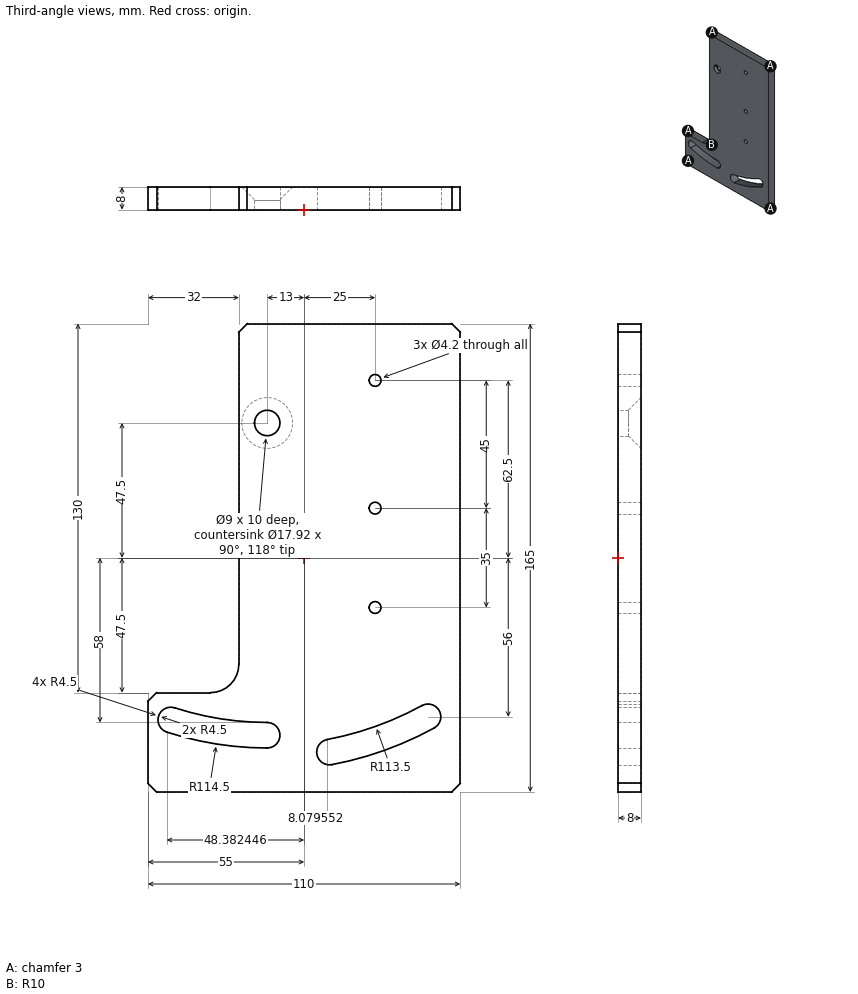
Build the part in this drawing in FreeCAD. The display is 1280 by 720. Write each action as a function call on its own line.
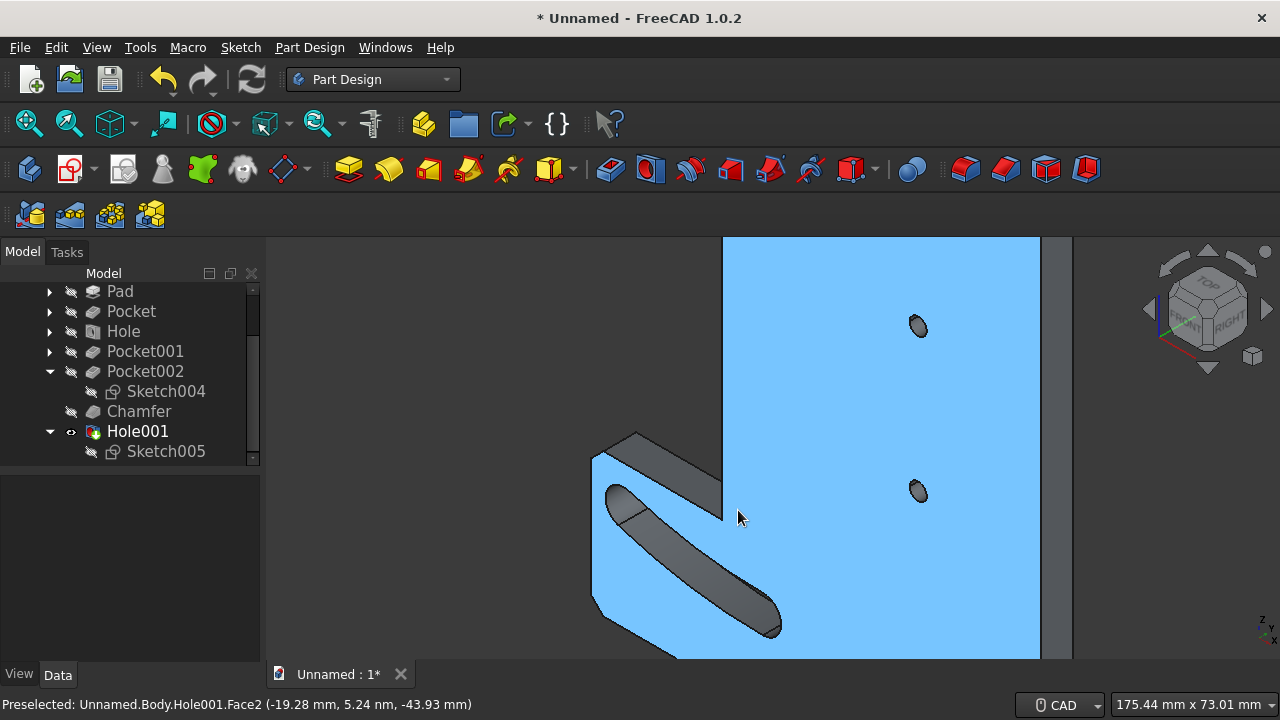
click(30, 124)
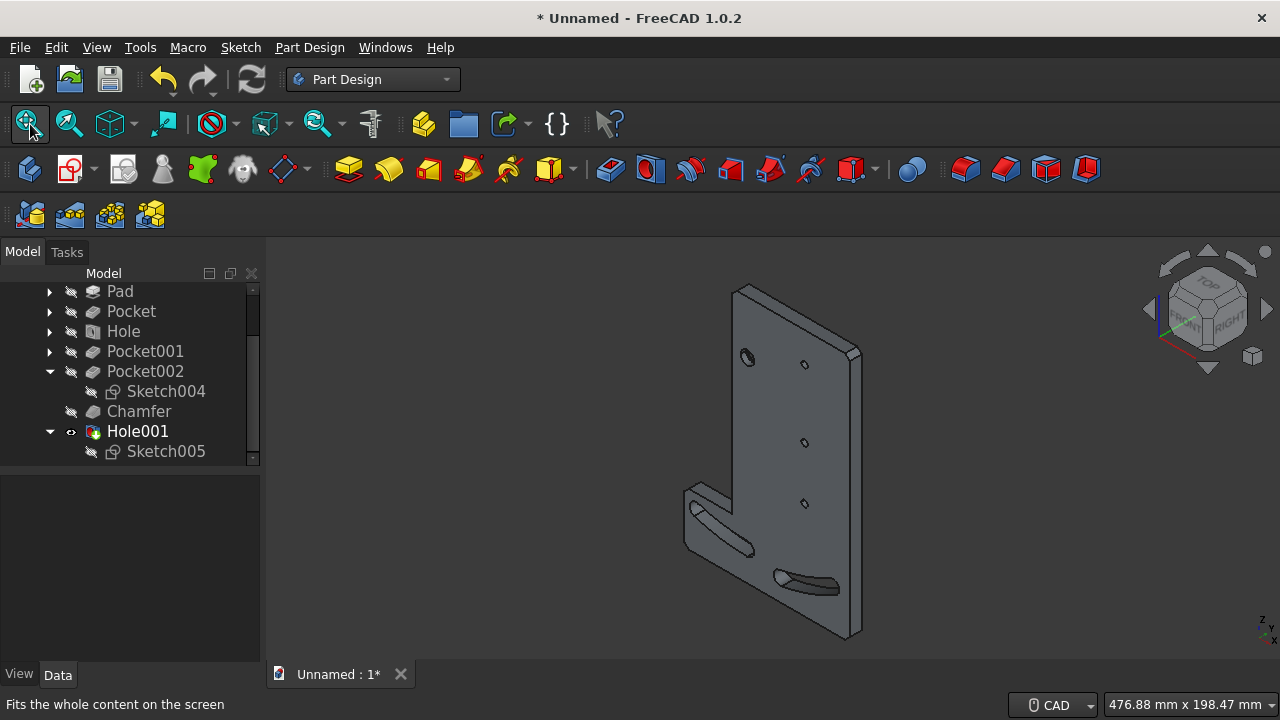
key(2)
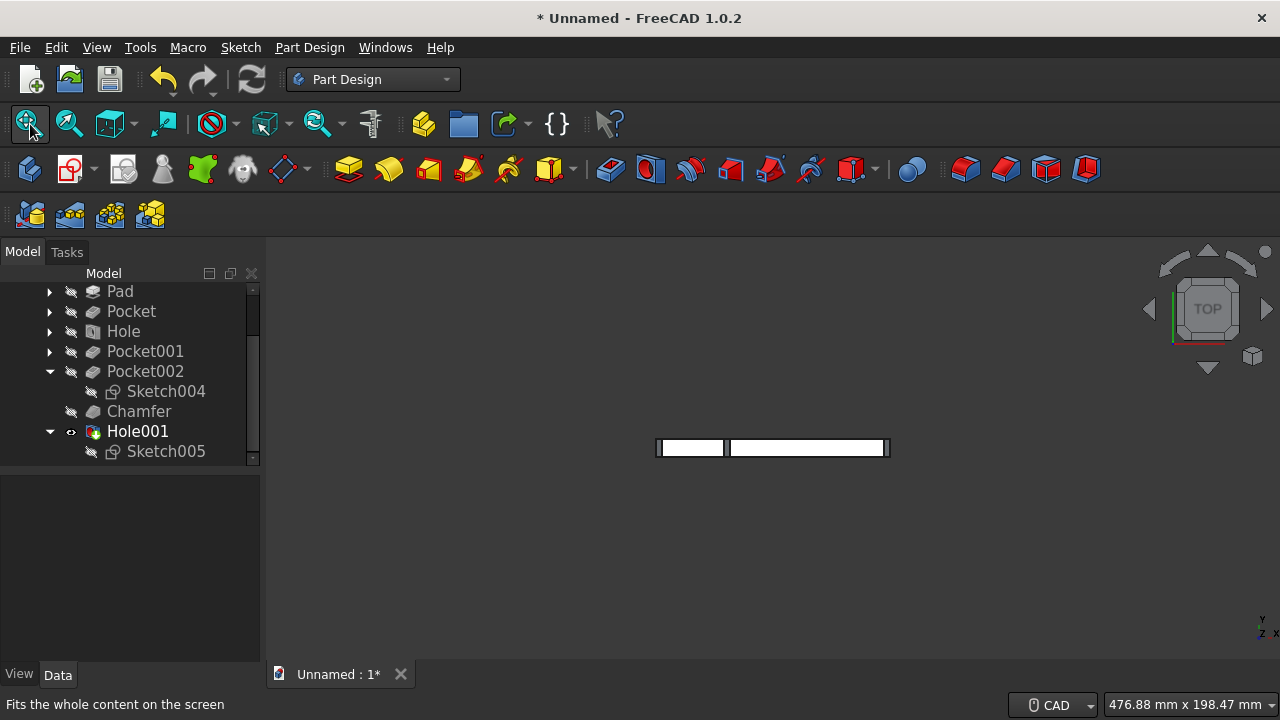
click(30, 124)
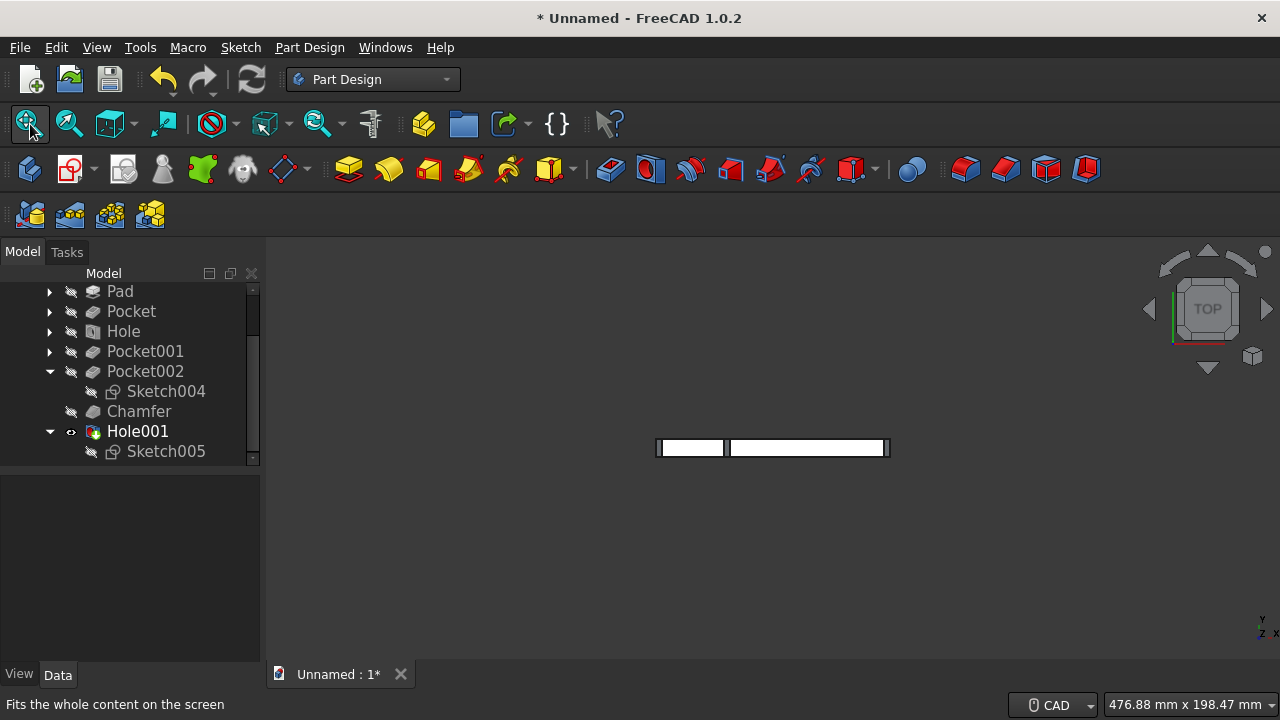
scroll(724, 447, up, 5)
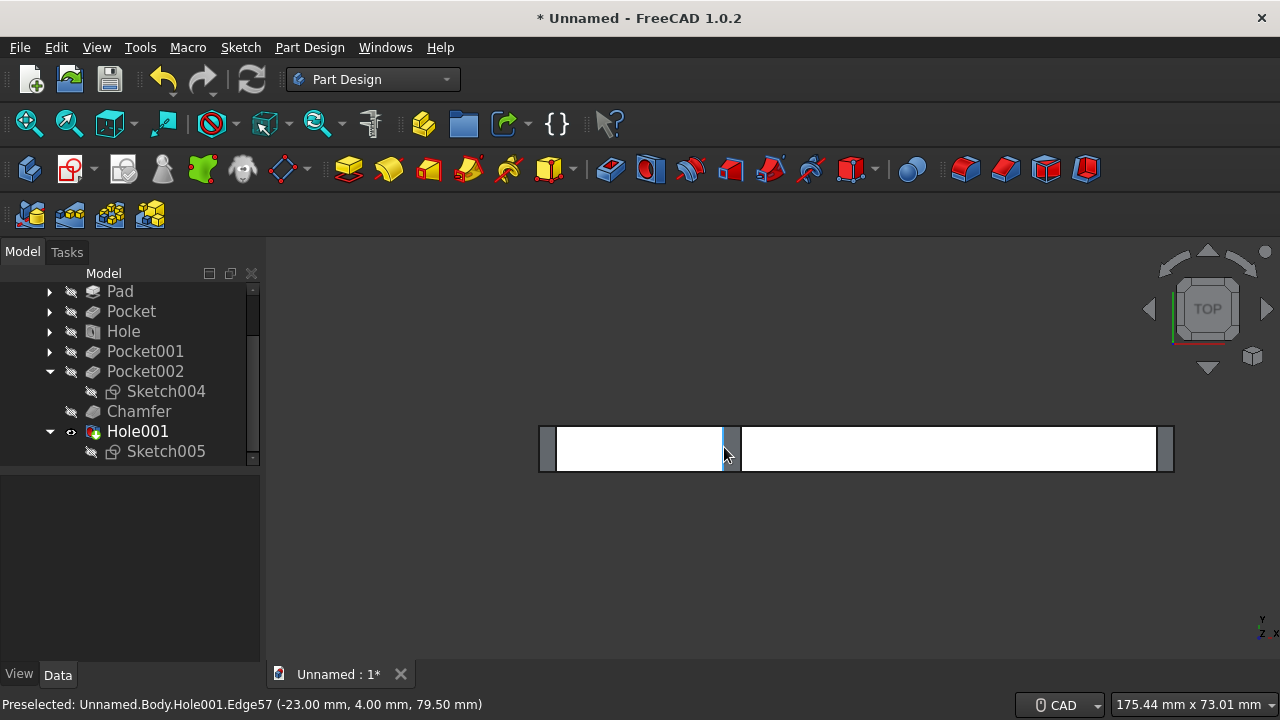
click(30, 124)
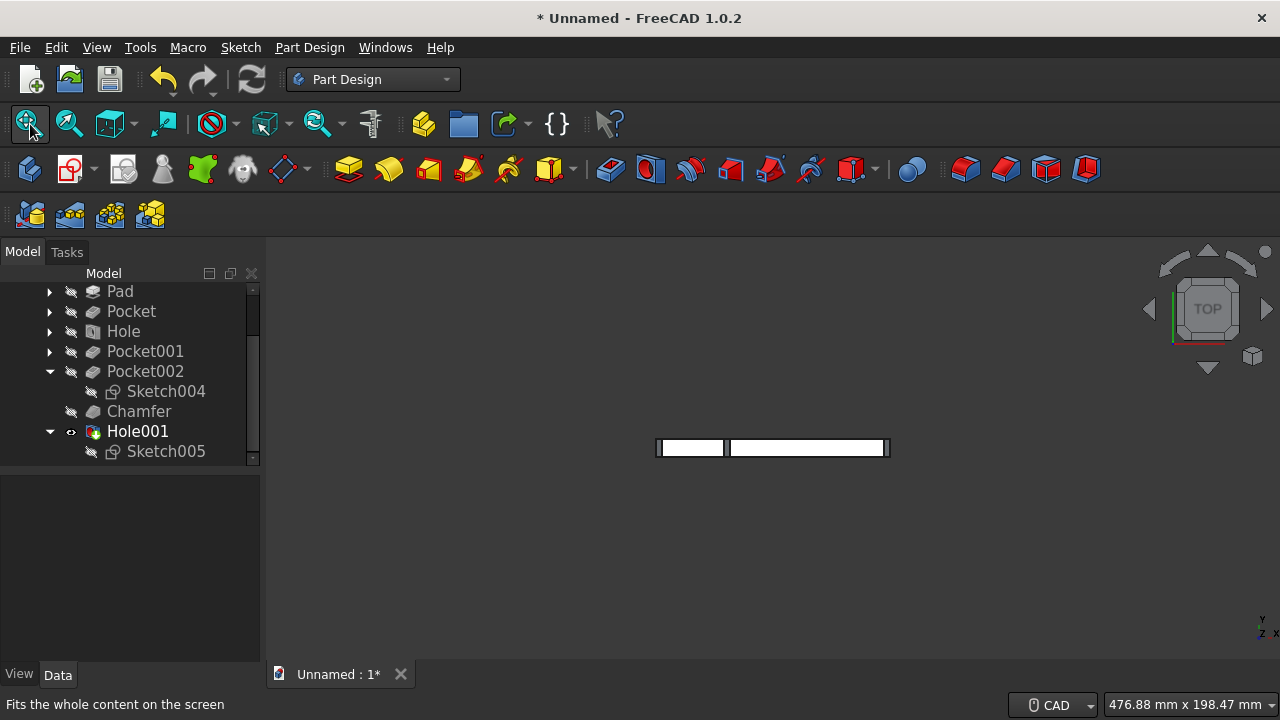
key(1)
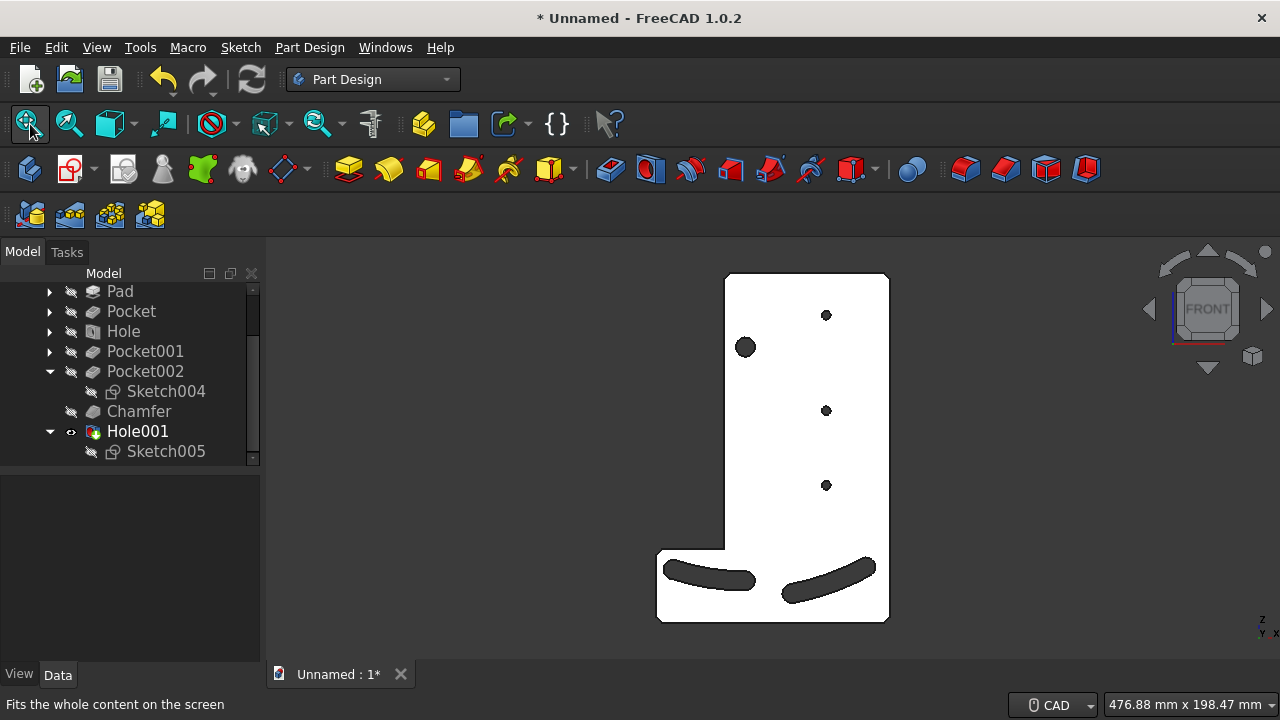
scroll(724, 548, up, 5)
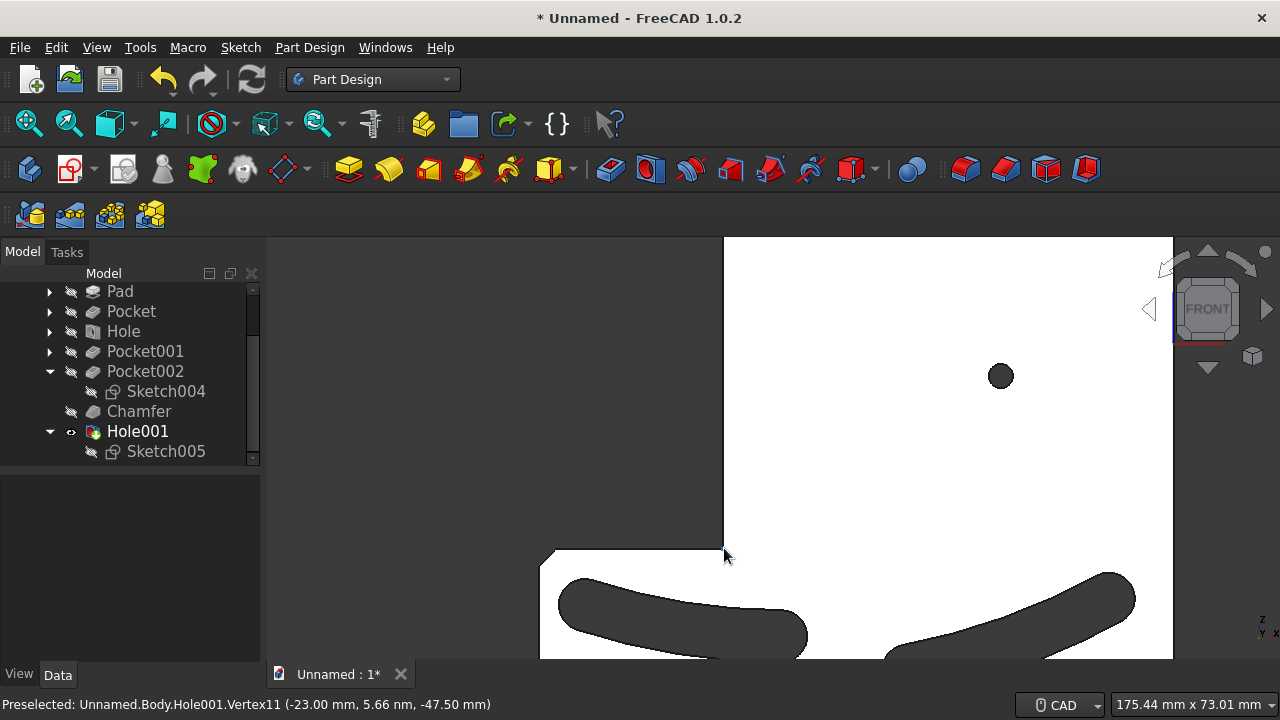
click(30, 124)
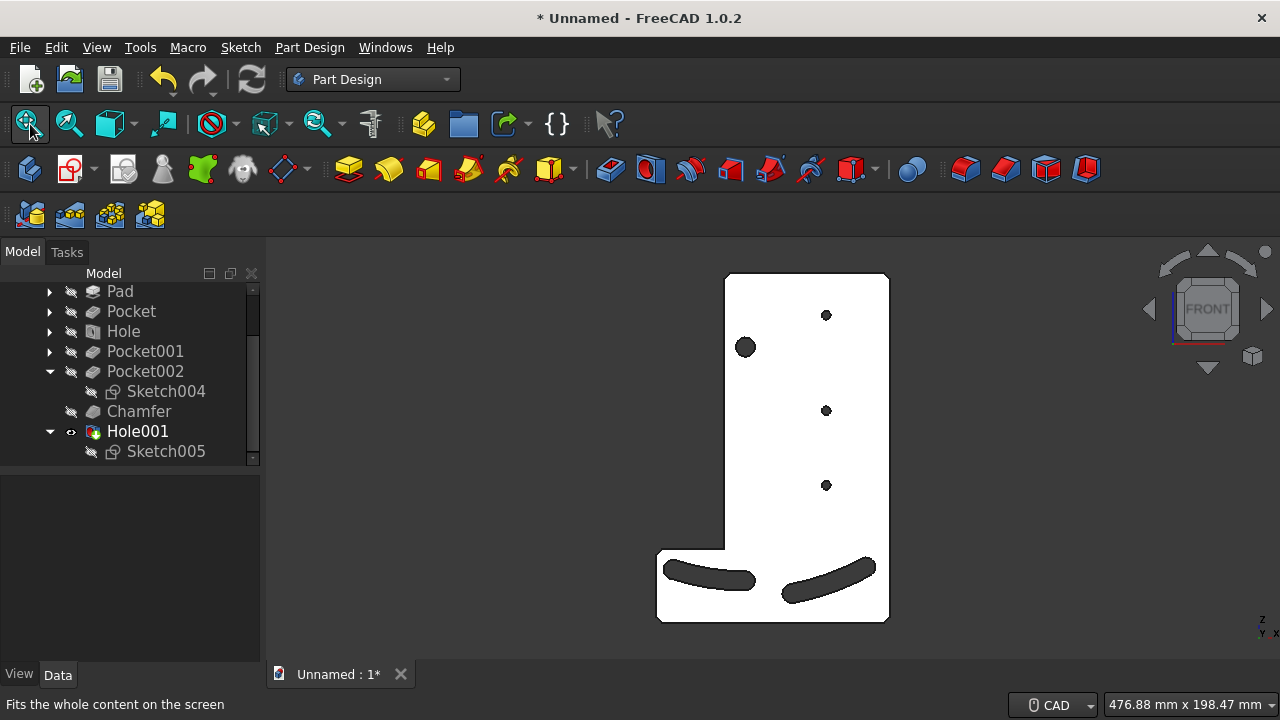
key(3)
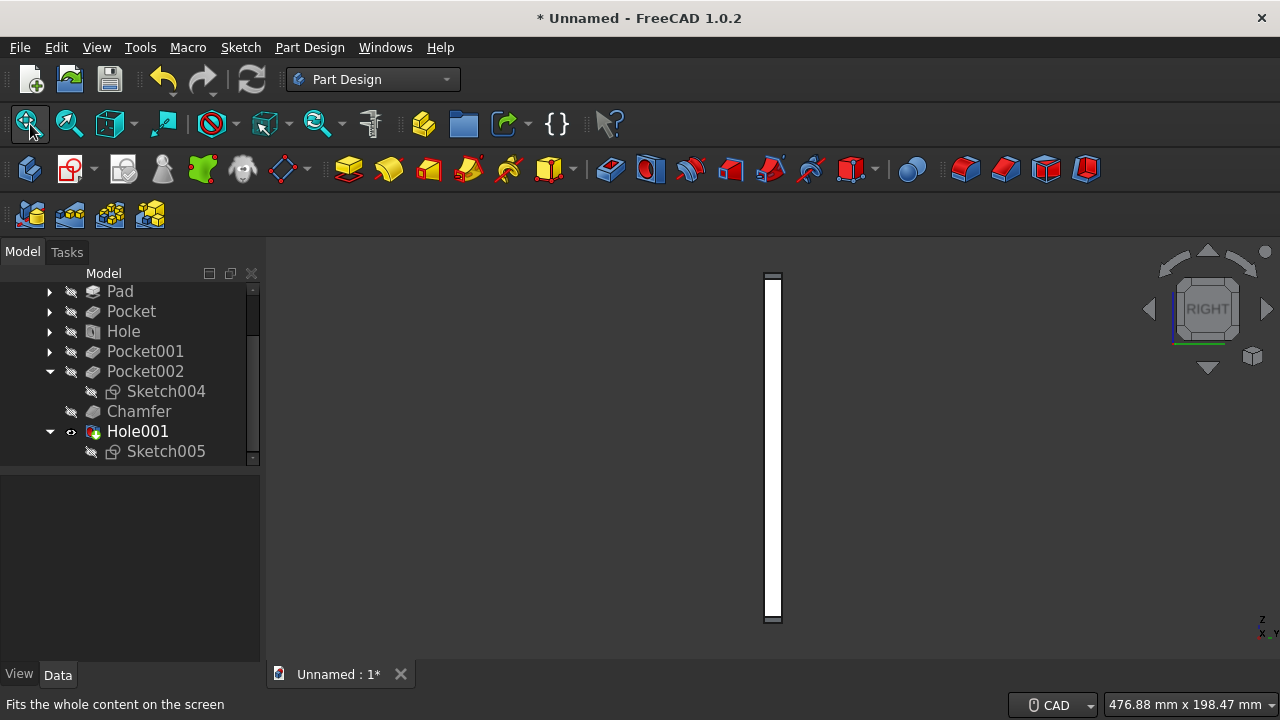
scroll(773, 548, up, 5)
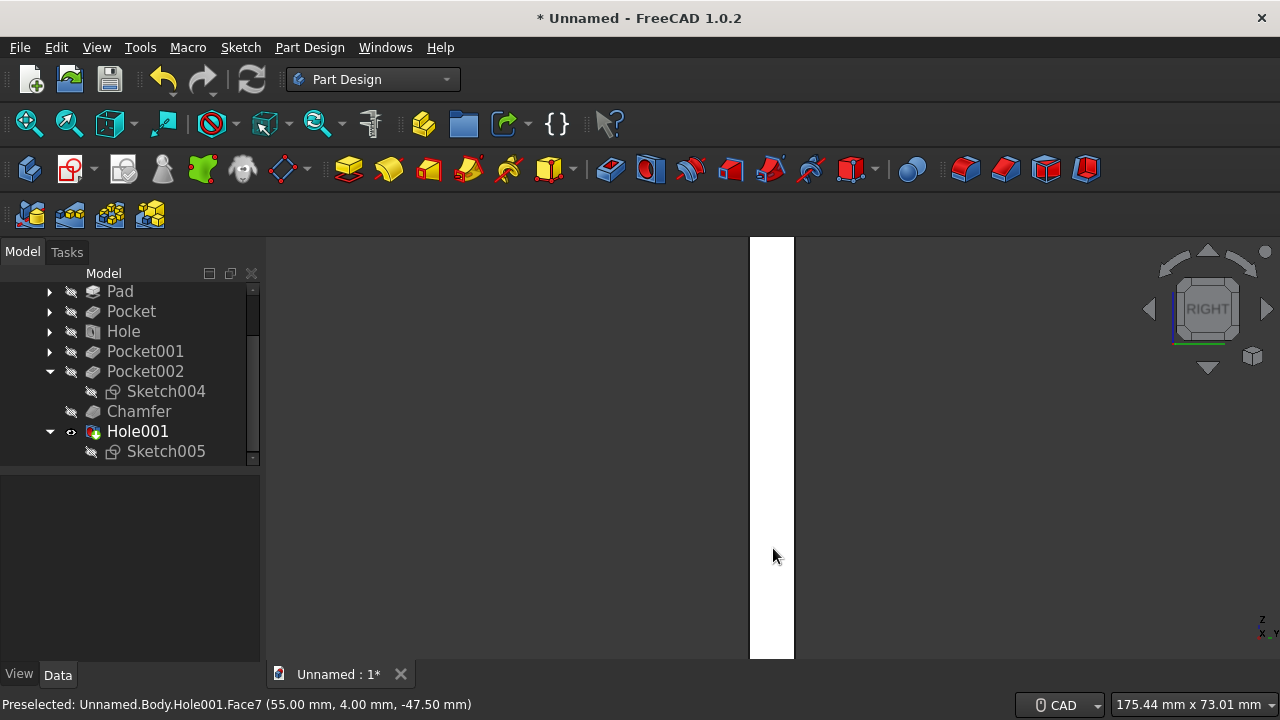
click(30, 124)